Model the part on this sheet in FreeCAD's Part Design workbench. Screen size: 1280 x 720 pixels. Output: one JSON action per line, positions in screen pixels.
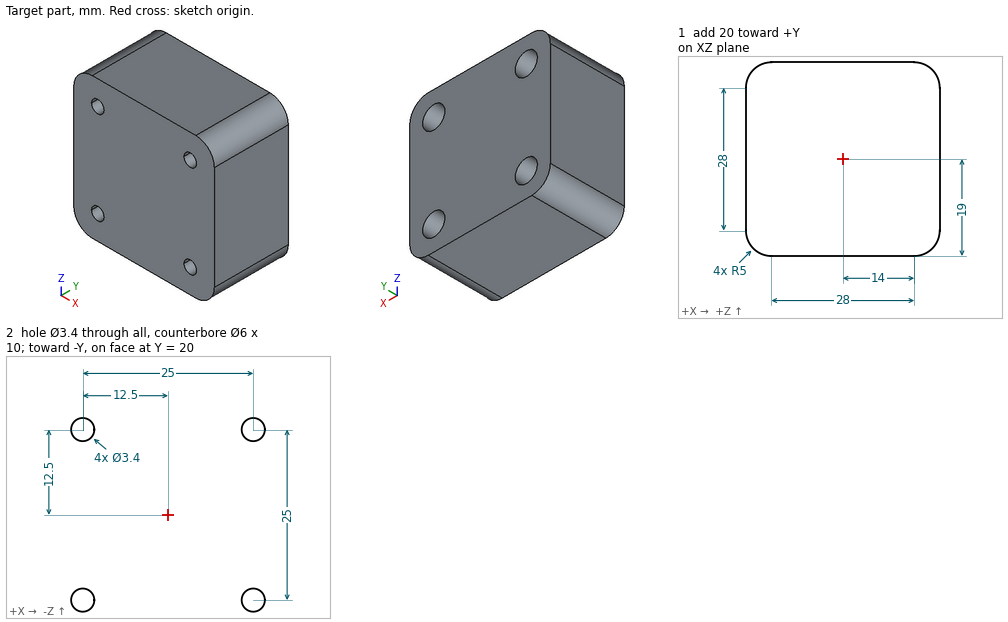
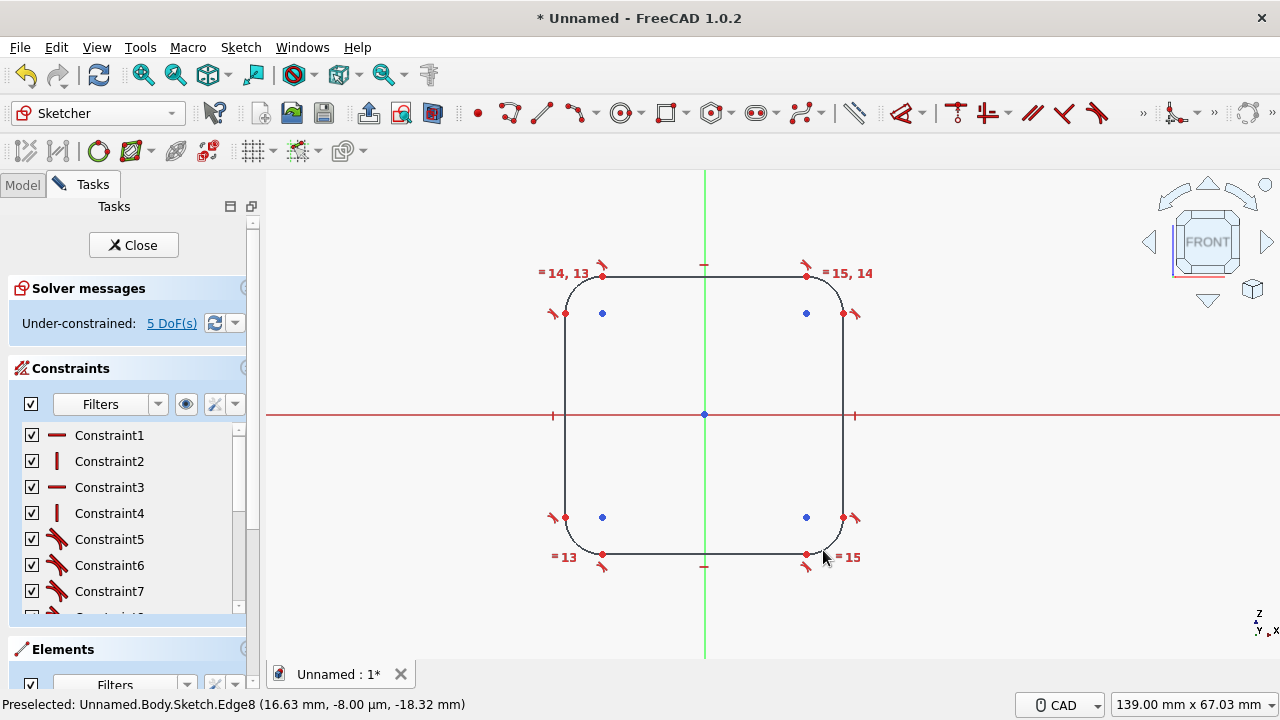
{"action": "left_click", "coordinate": [902, 114]}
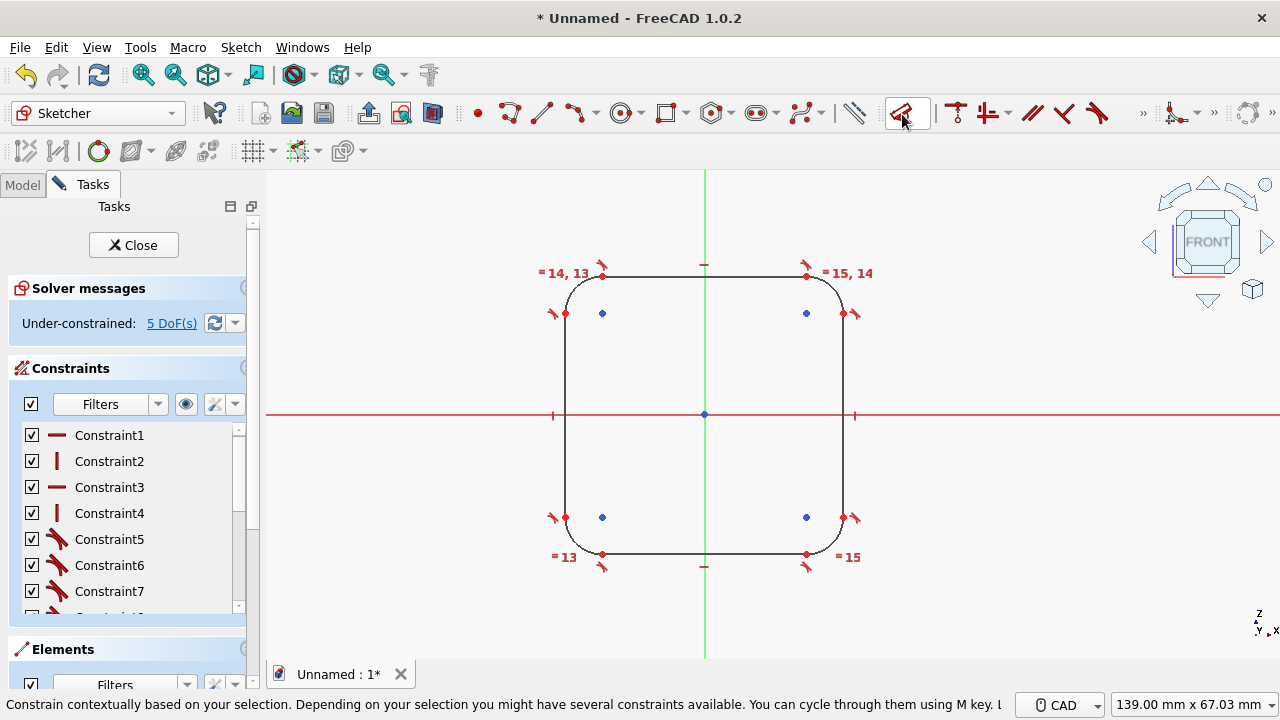
{"action": "left_click", "coordinate": [569, 534]}
{"action": "left_click", "coordinate": [540, 548]}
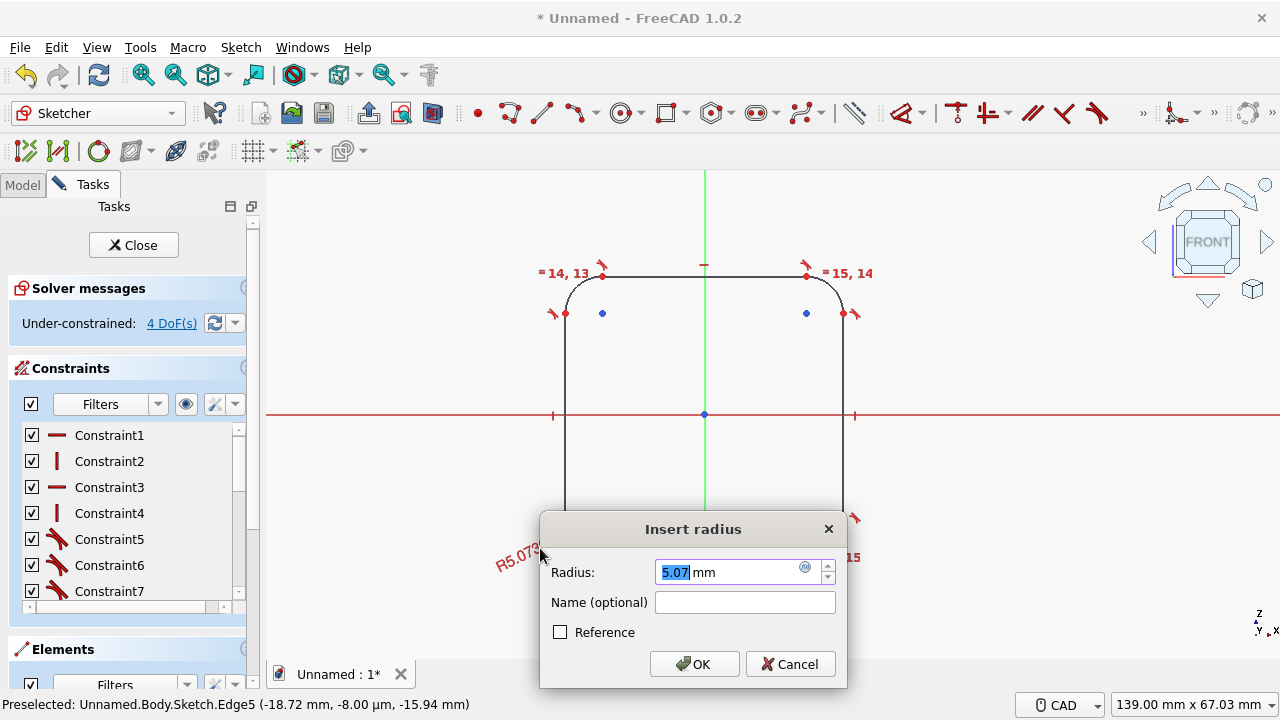
{"action": "type", "text": "5"}
{"action": "key", "text": "Return"}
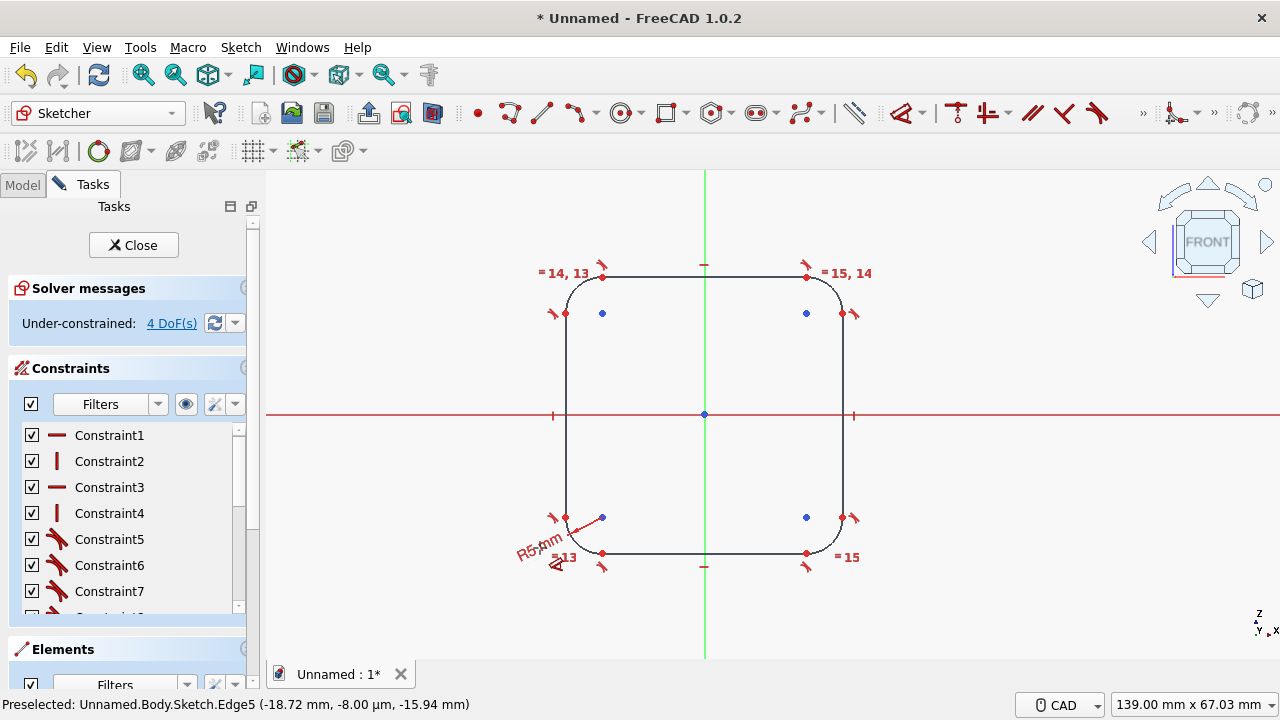
{"action": "left_click", "coordinate": [745, 554]}
{"action": "left_click", "coordinate": [657, 588]}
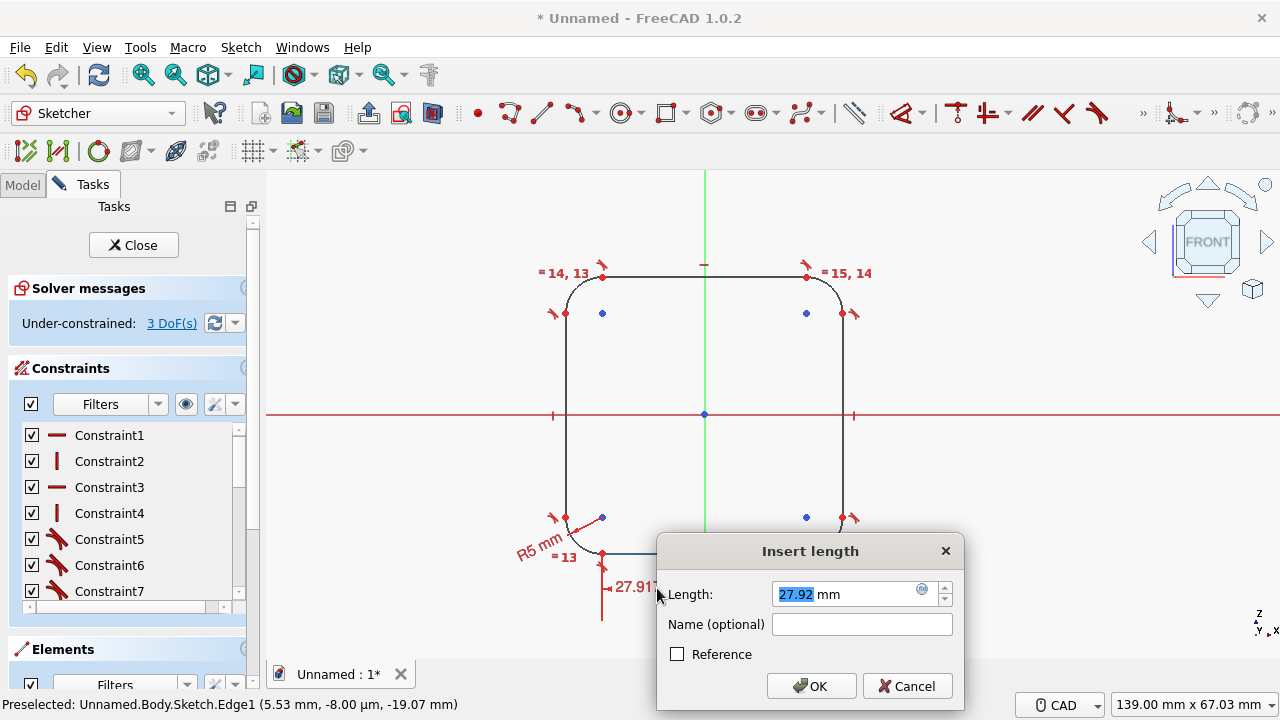
{"action": "type", "text": "28"}
{"action": "key", "text": "Return"}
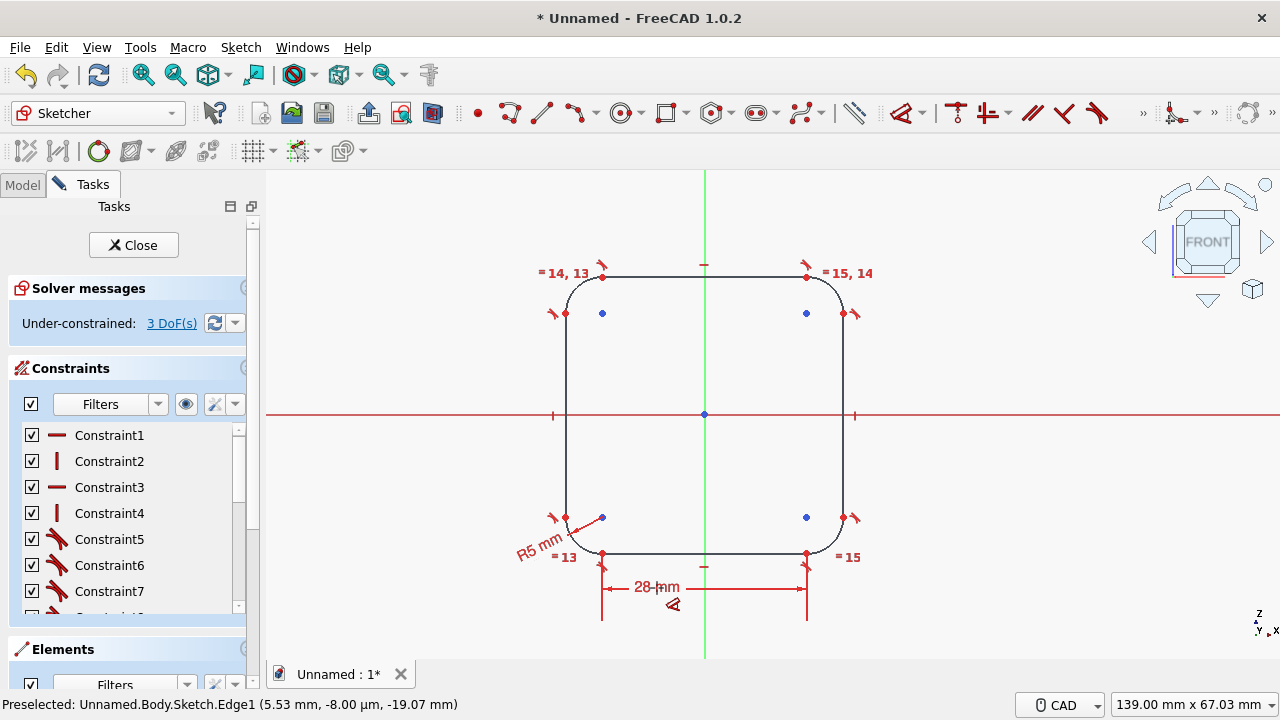
{"action": "left_click", "coordinate": [566, 456]}
{"action": "left_click", "coordinate": [532, 369]}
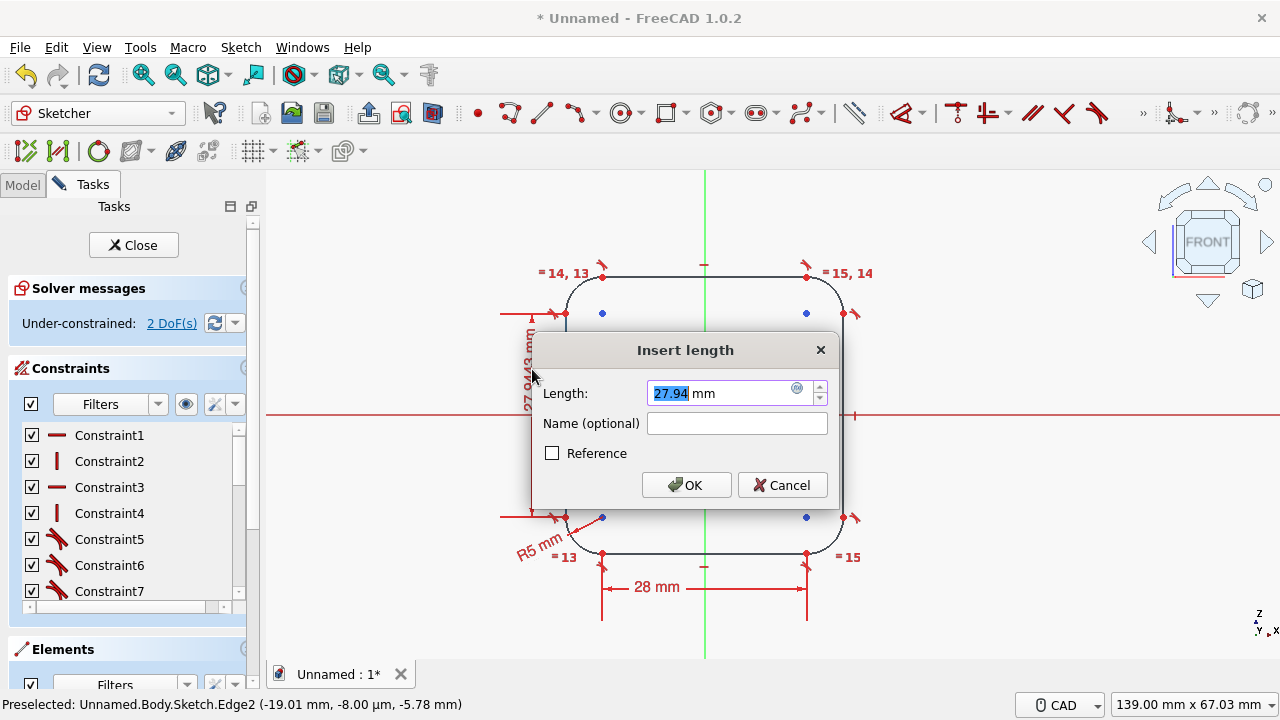
{"action": "type", "text": "28"}
{"action": "key", "text": "Return"}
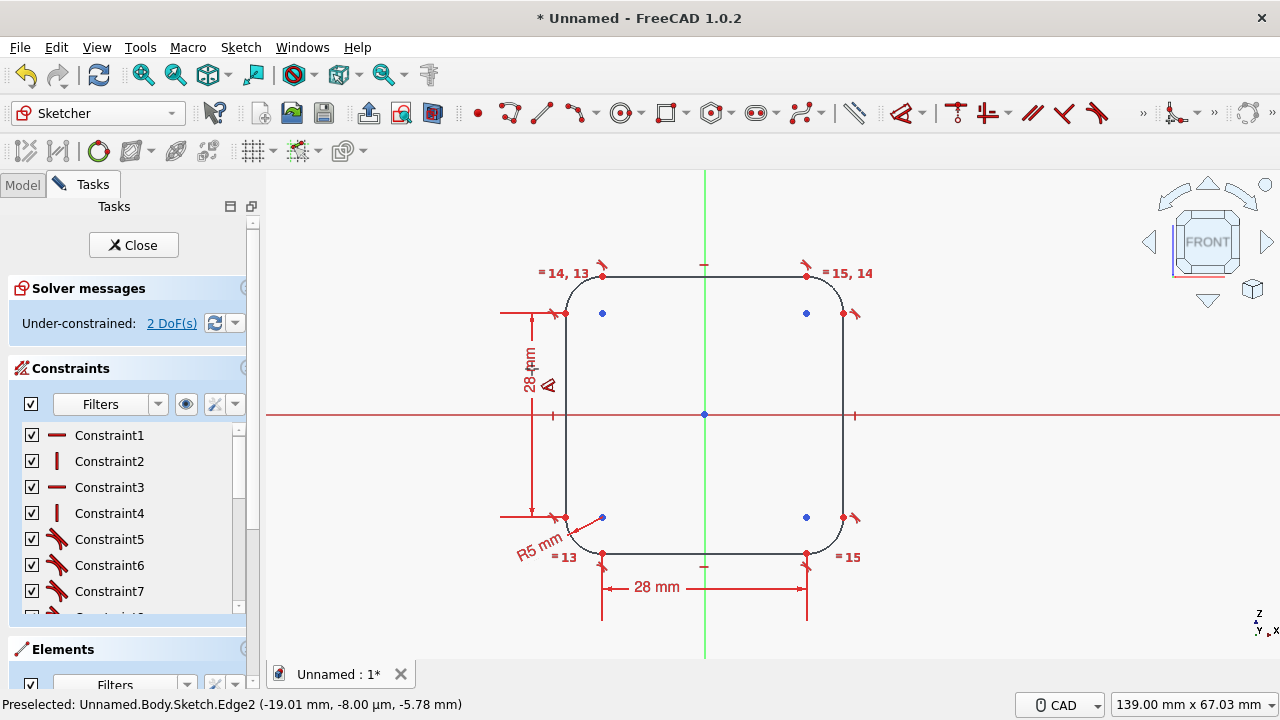
{"action": "left_click", "coordinate": [807, 554]}
{"action": "left_click", "coordinate": [756, 588]}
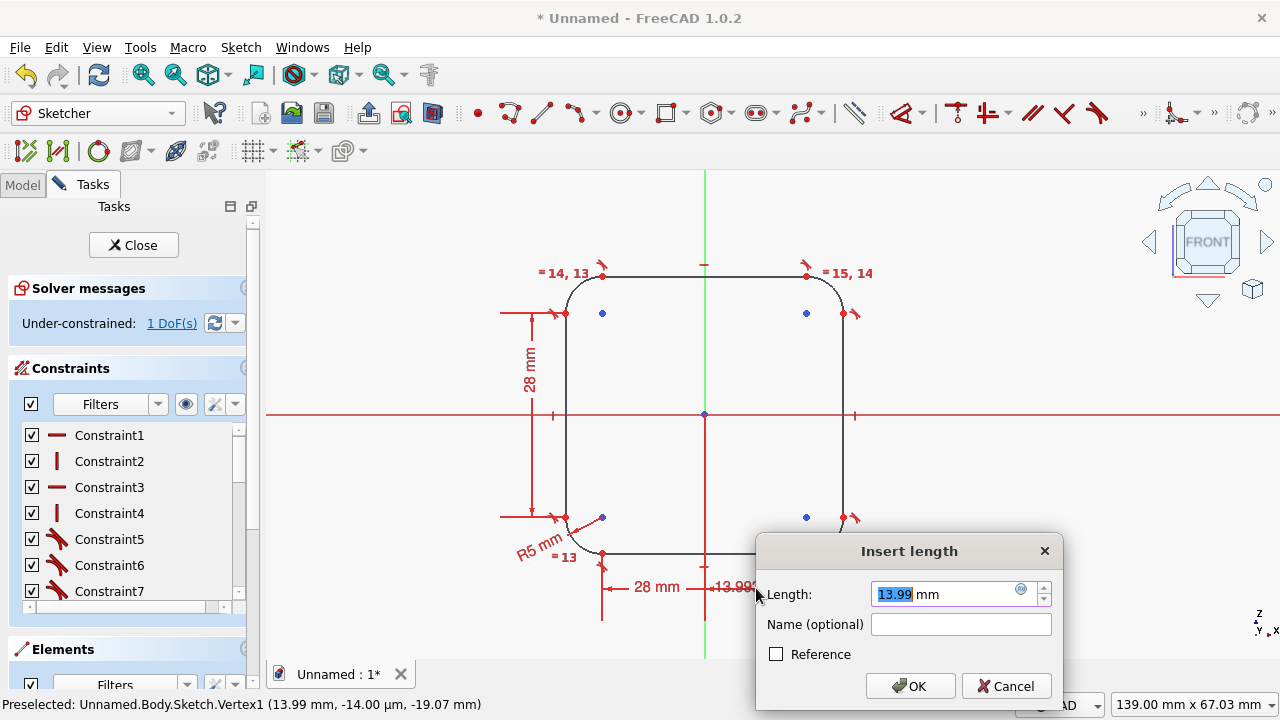
{"action": "type", "text": "14"}
{"action": "key", "text": "Return"}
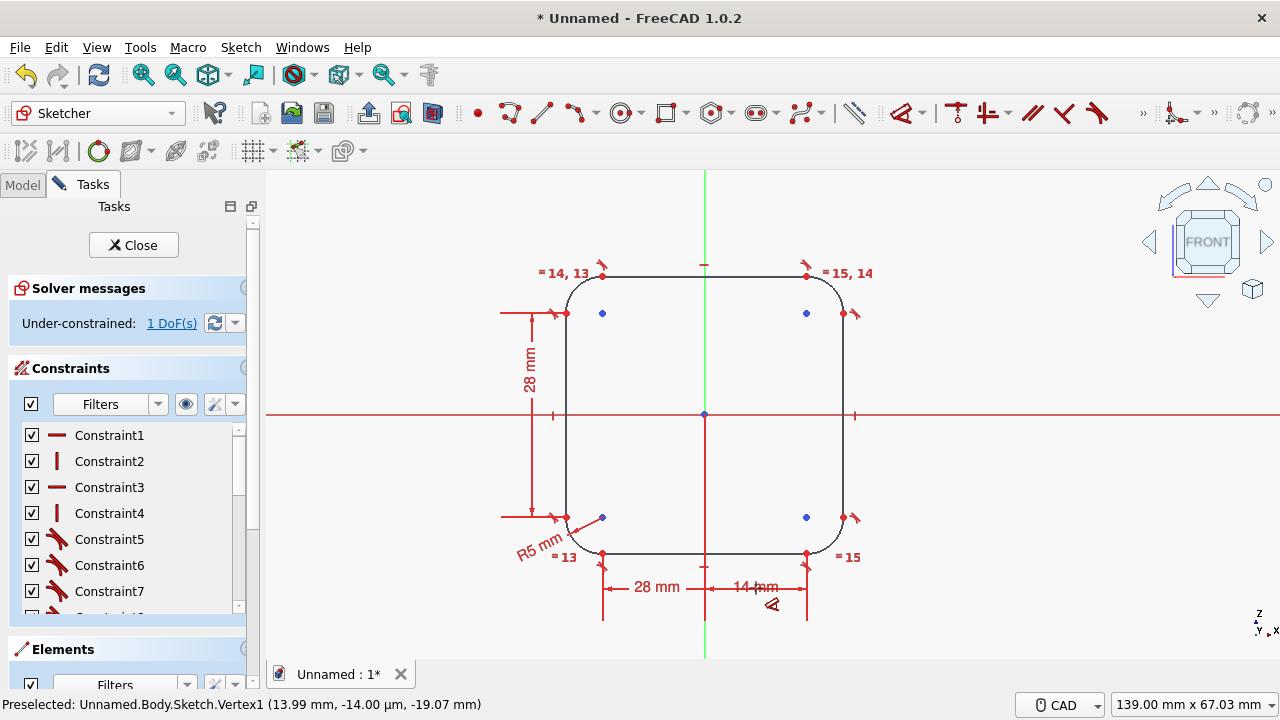
{"action": "left_click", "coordinate": [807, 554]}
{"action": "left_click", "coordinate": [671, 484]}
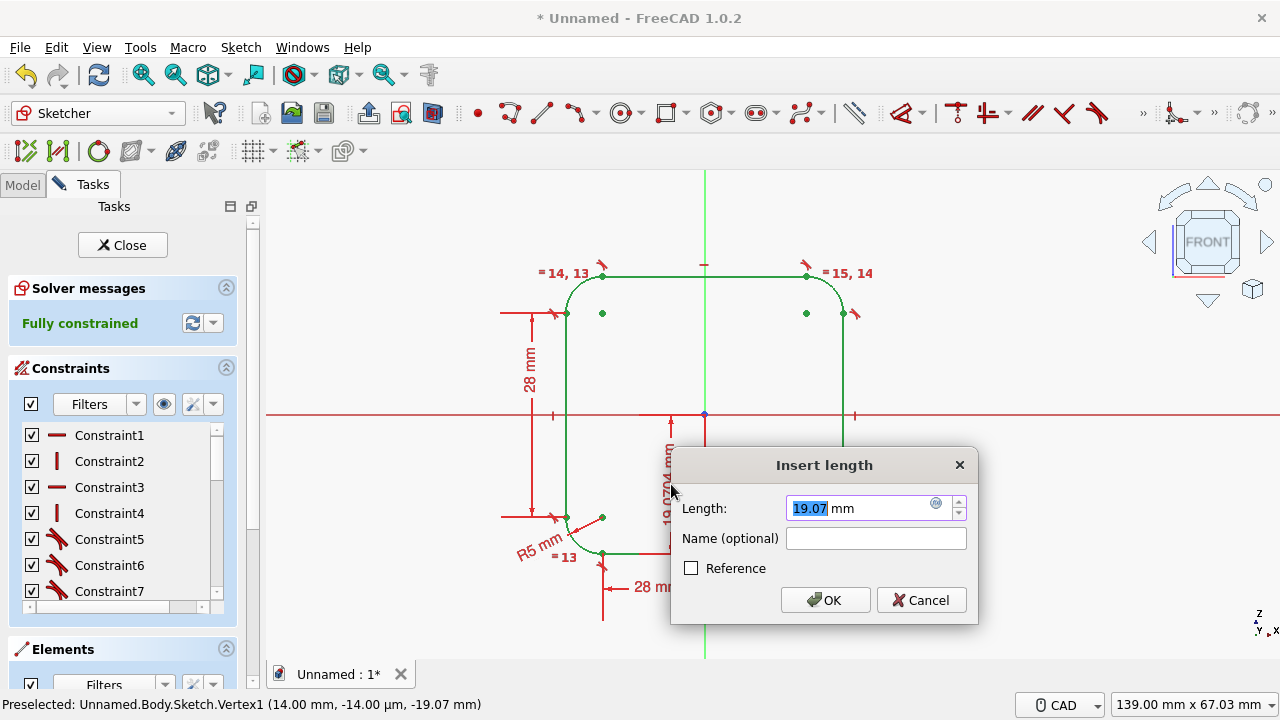
{"action": "type", "text": "19"}
{"action": "key", "text": "Return"}
{"action": "key", "text": "Escape"}